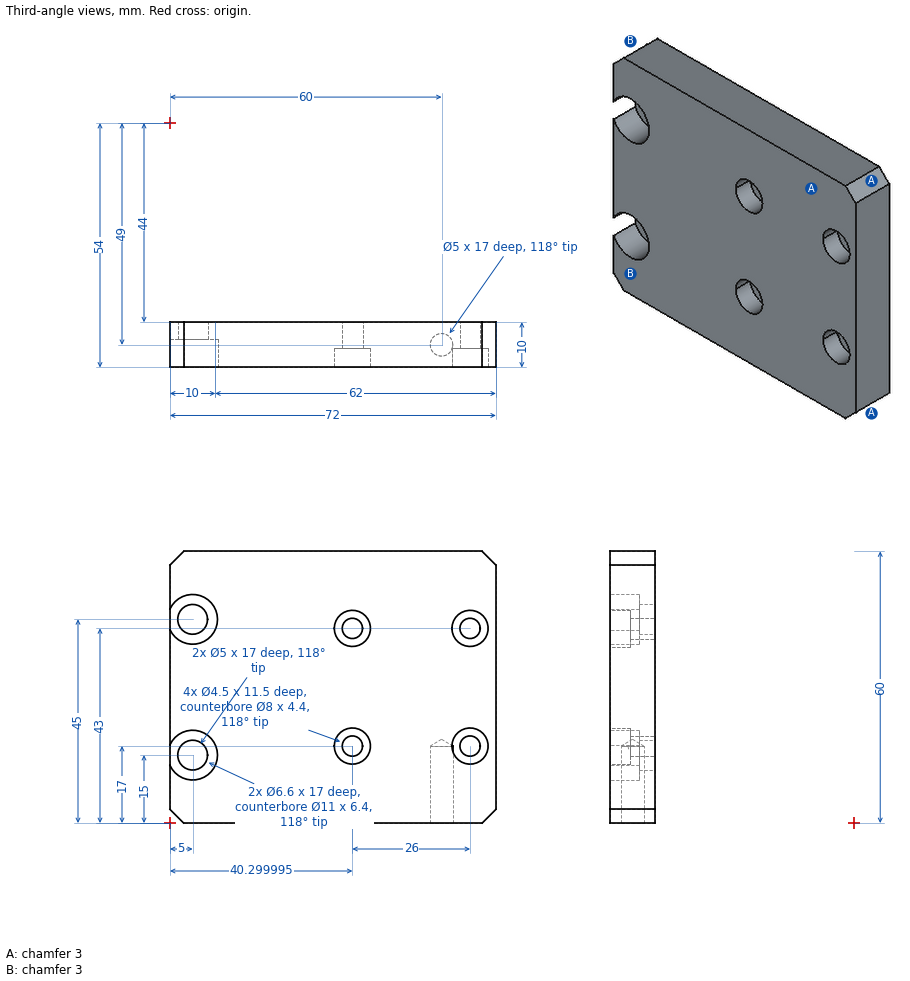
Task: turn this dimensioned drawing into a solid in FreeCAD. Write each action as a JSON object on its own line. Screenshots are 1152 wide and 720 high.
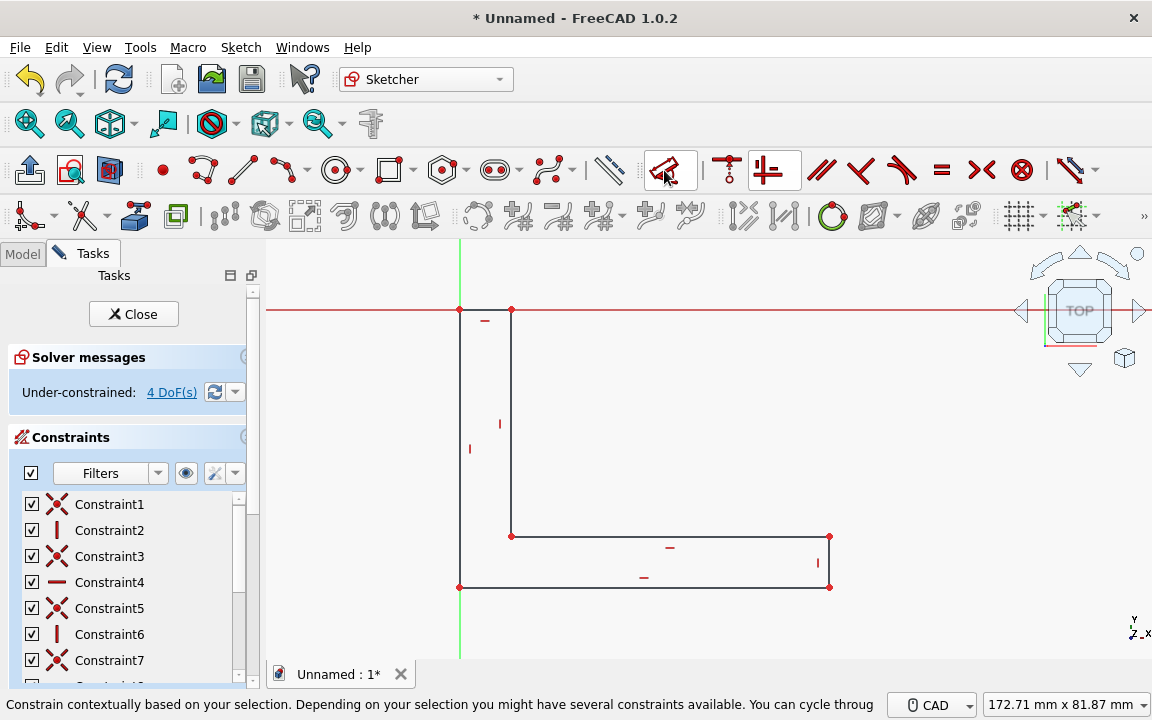
{"action": "left_click", "coordinate": [460, 393]}
{"action": "left_click", "coordinate": [426, 449]}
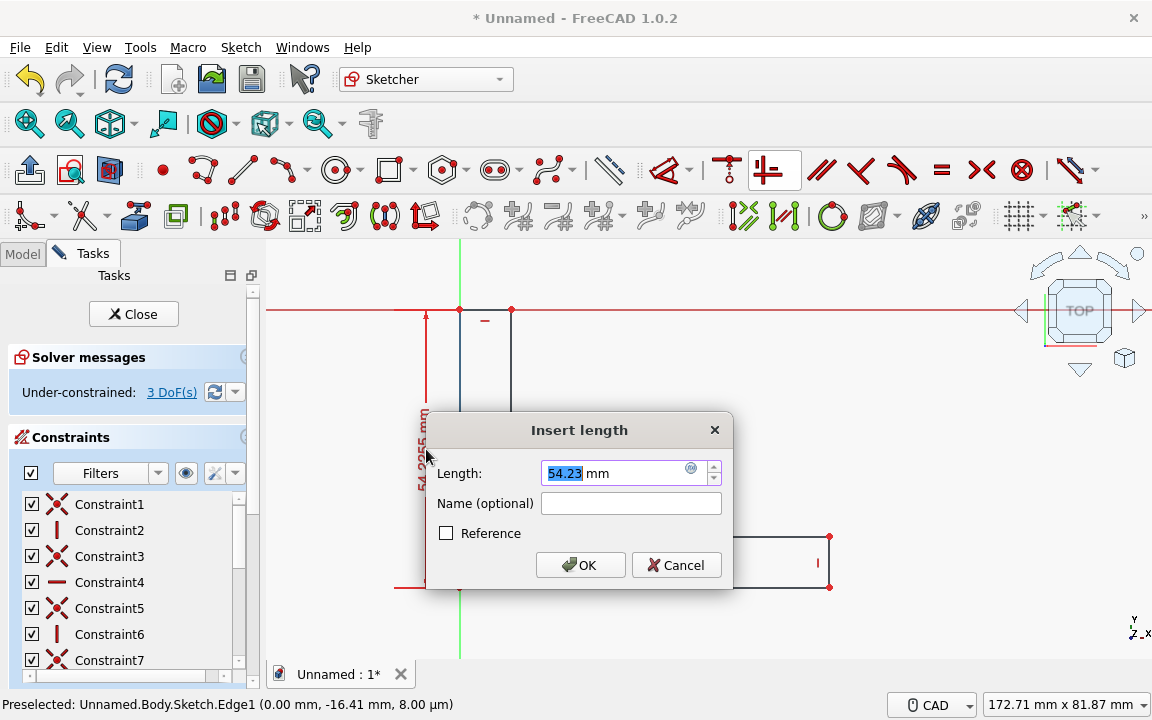
{"action": "type", "text": "54"}
{"action": "key", "text": "Return"}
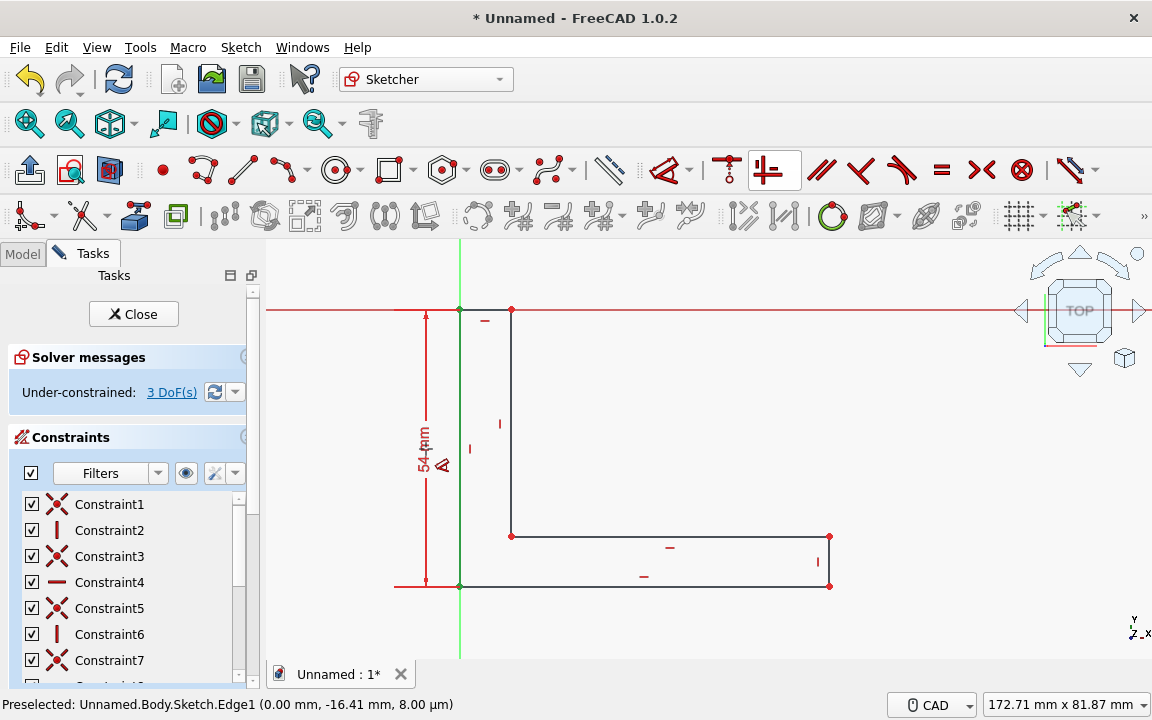
{"action": "left_click", "coordinate": [570, 587]}
{"action": "left_click", "coordinate": [644, 621]}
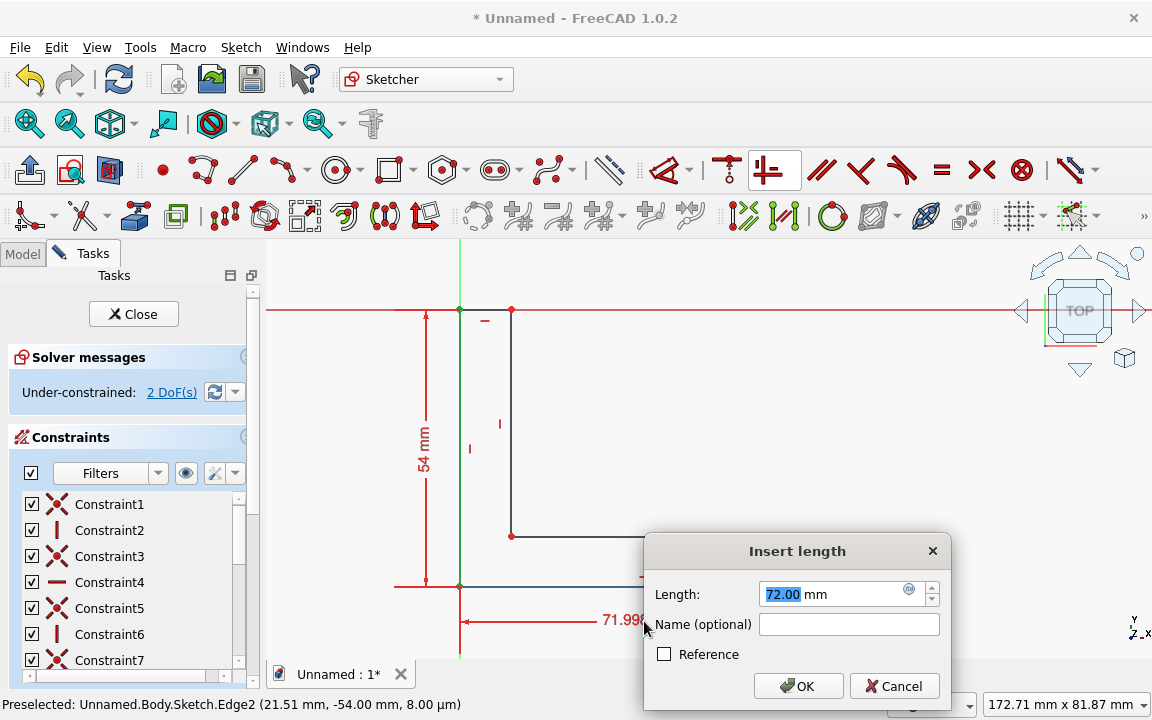
{"action": "type", "text": "72"}
{"action": "key", "text": "Return"}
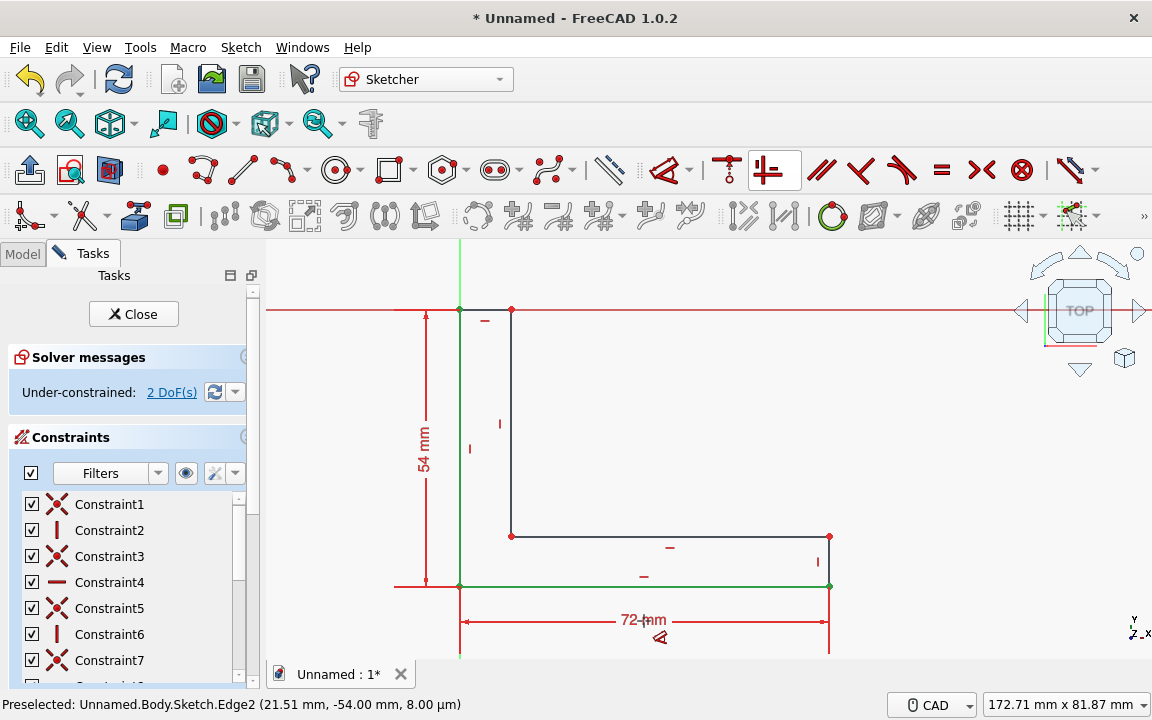
{"action": "left_click", "coordinate": [829, 572]}
{"action": "left_click", "coordinate": [863, 562]}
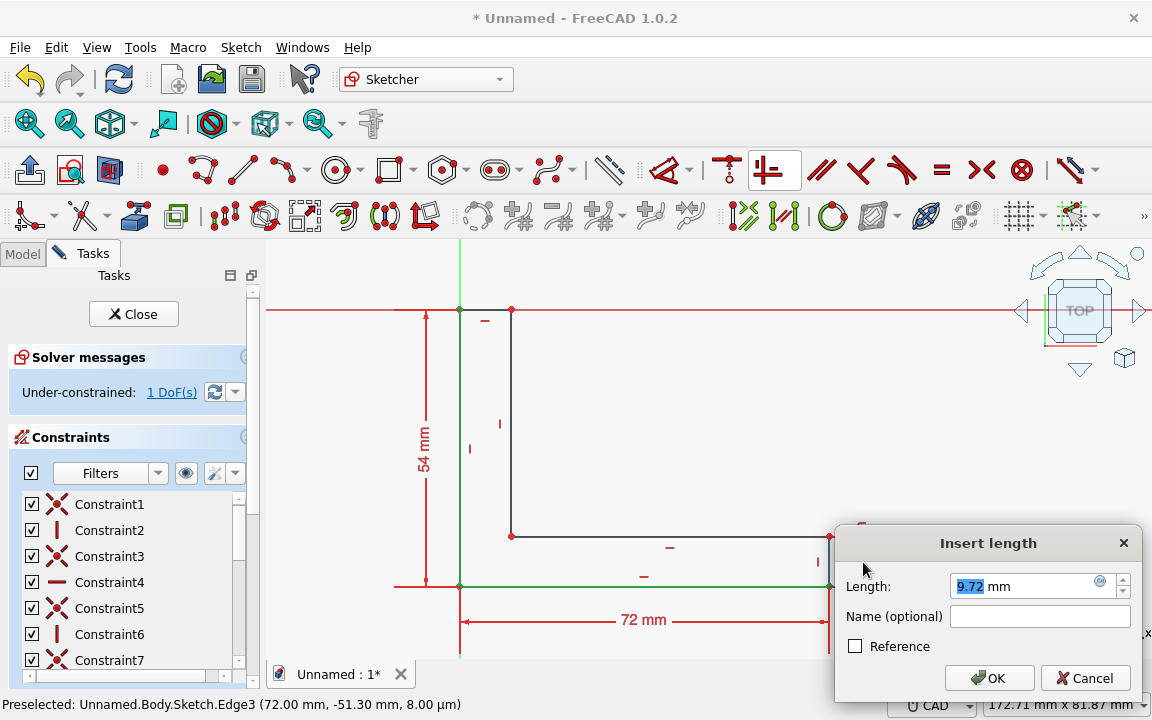
{"action": "type", "text": "10"}
{"action": "key", "text": "Return"}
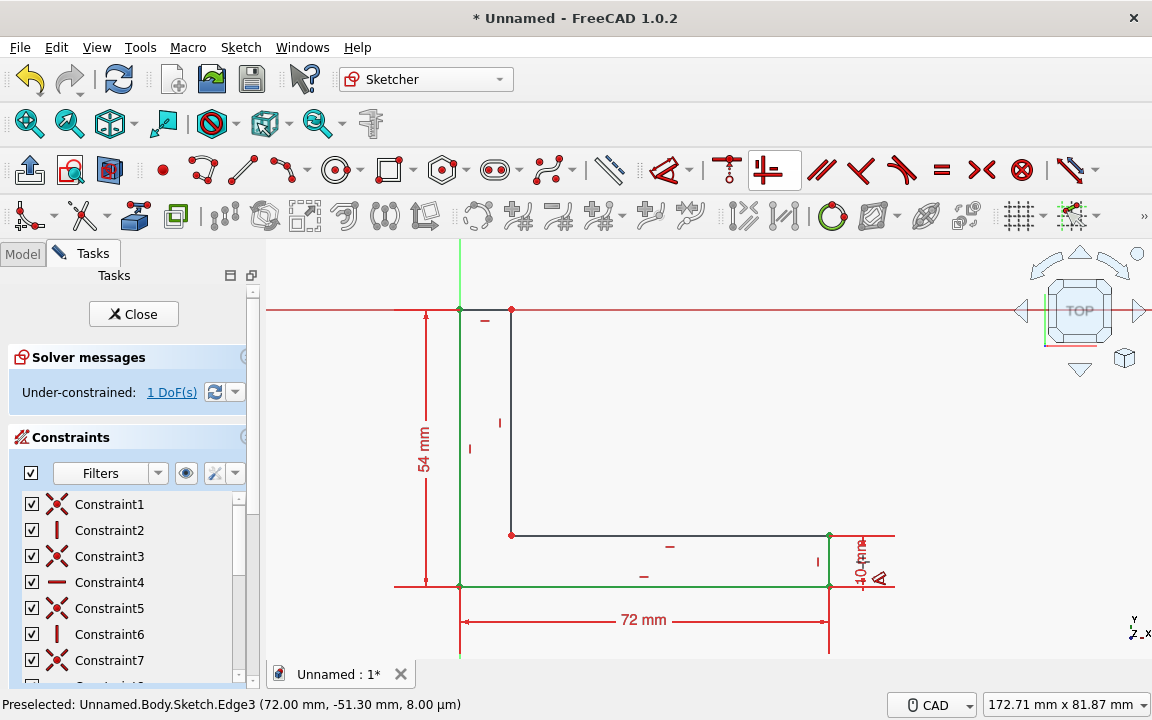
{"action": "left_click", "coordinate": [734, 536]}
{"action": "left_click", "coordinate": [670, 570]}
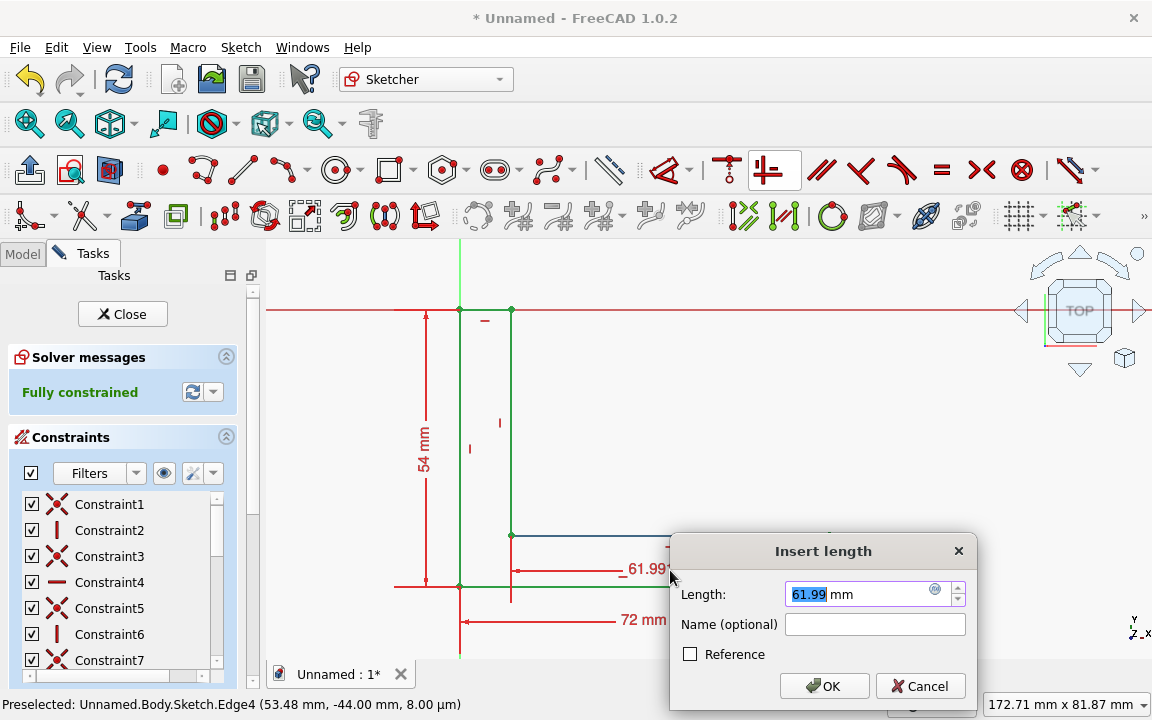
{"action": "type", "text": "62"}
{"action": "key", "text": "Return"}
{"action": "key", "text": "Escape"}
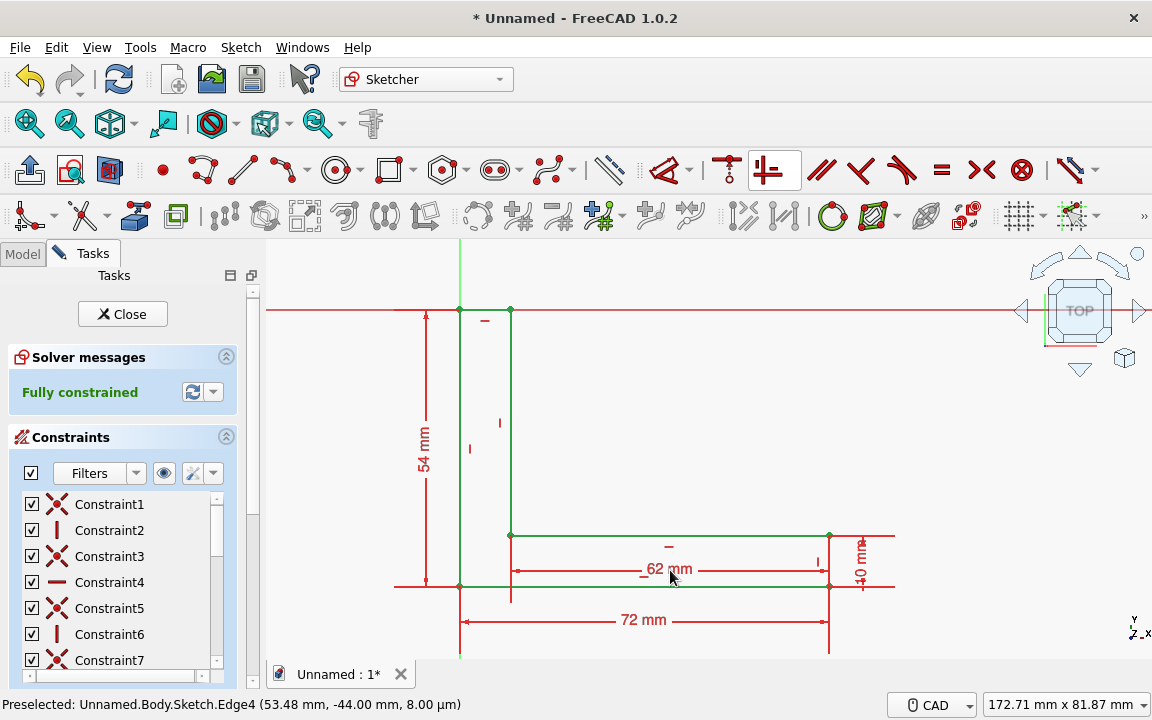
{"action": "left_click", "coordinate": [123, 314]}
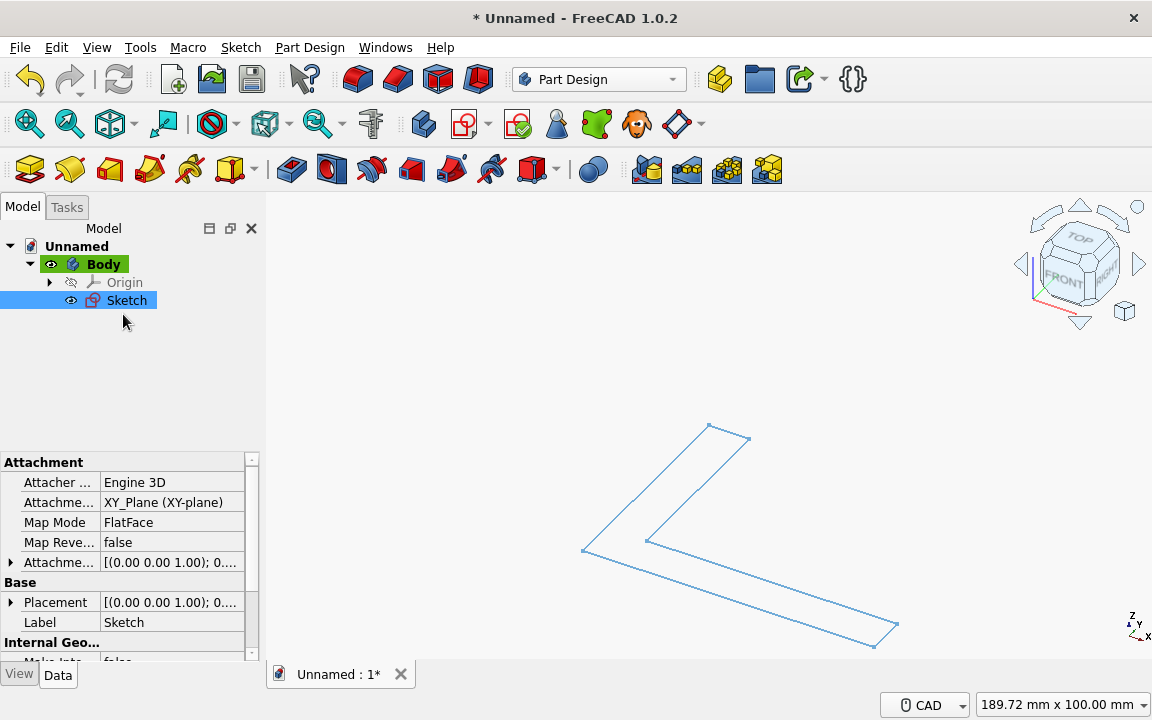
{"action": "left_click", "coordinate": [30, 170]}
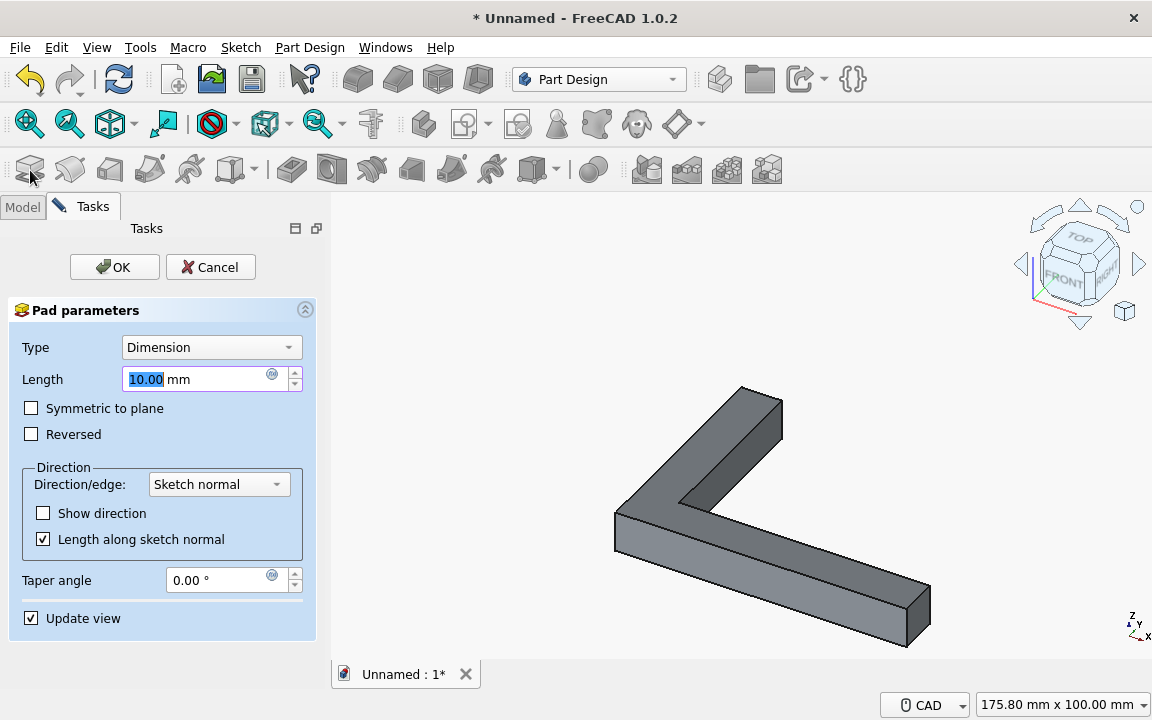
{"action": "type", "text": "60"}
{"action": "key", "text": "Tab"}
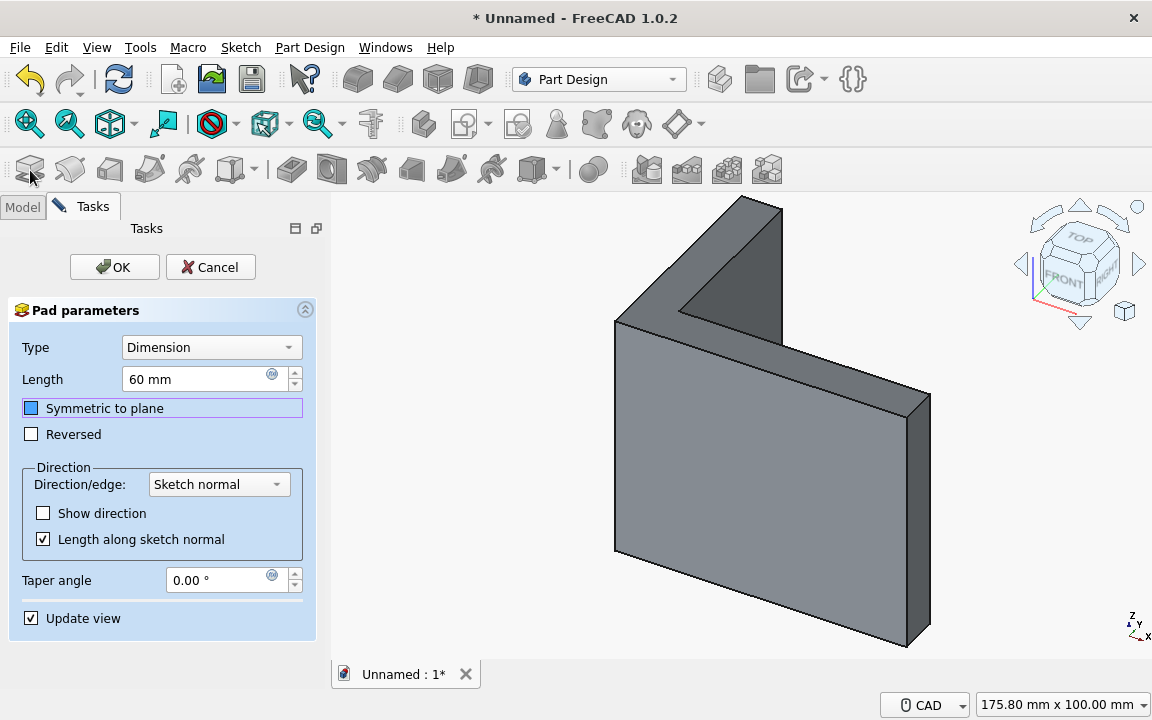
{"action": "left_click", "coordinate": [115, 267]}